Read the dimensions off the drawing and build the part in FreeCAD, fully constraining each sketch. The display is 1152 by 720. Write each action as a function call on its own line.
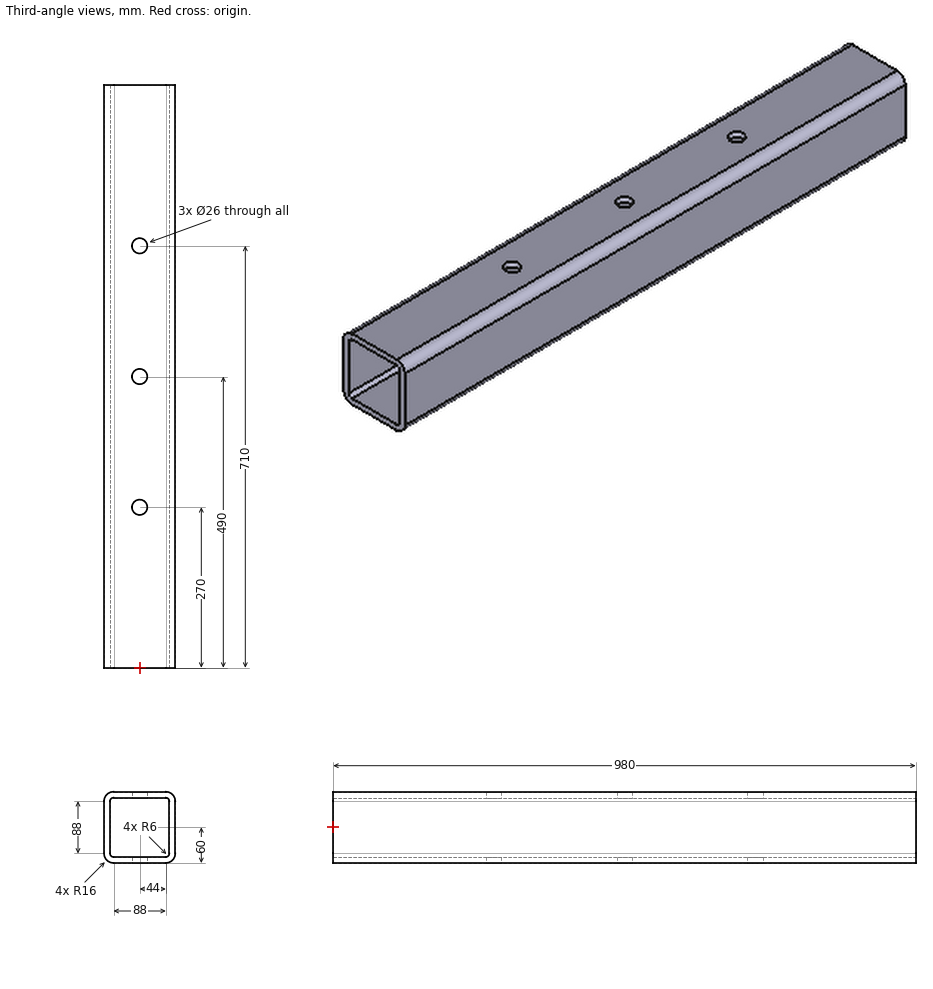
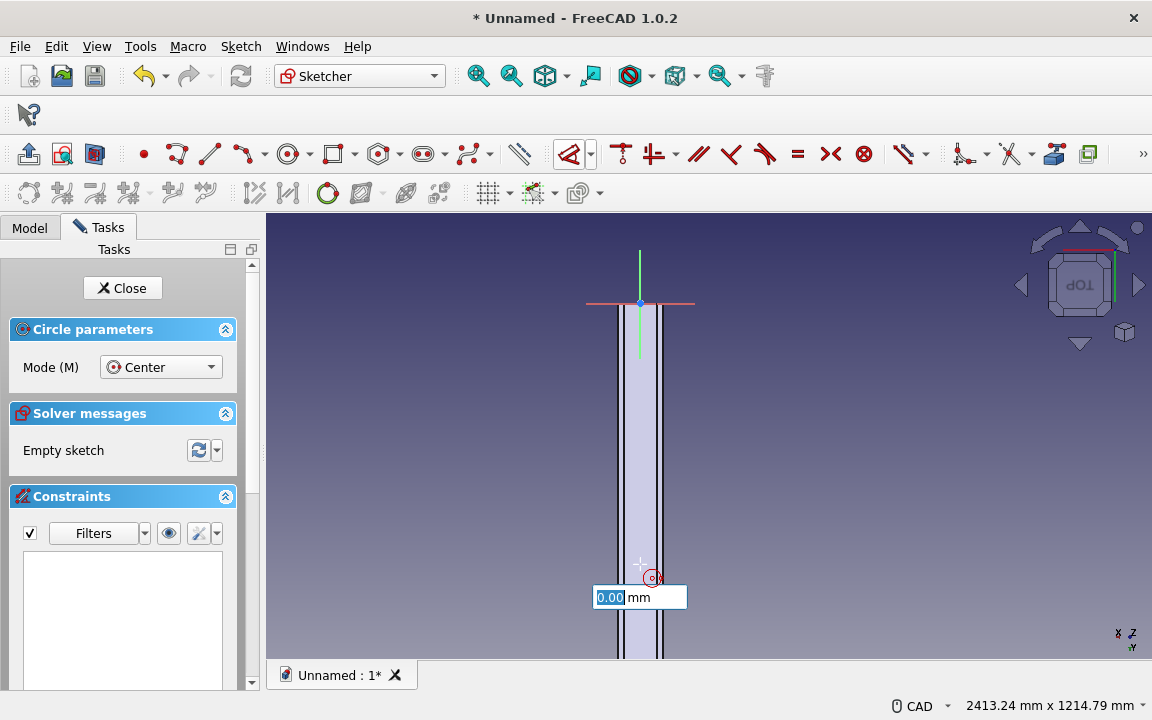
scroll(645, 563, up, 7)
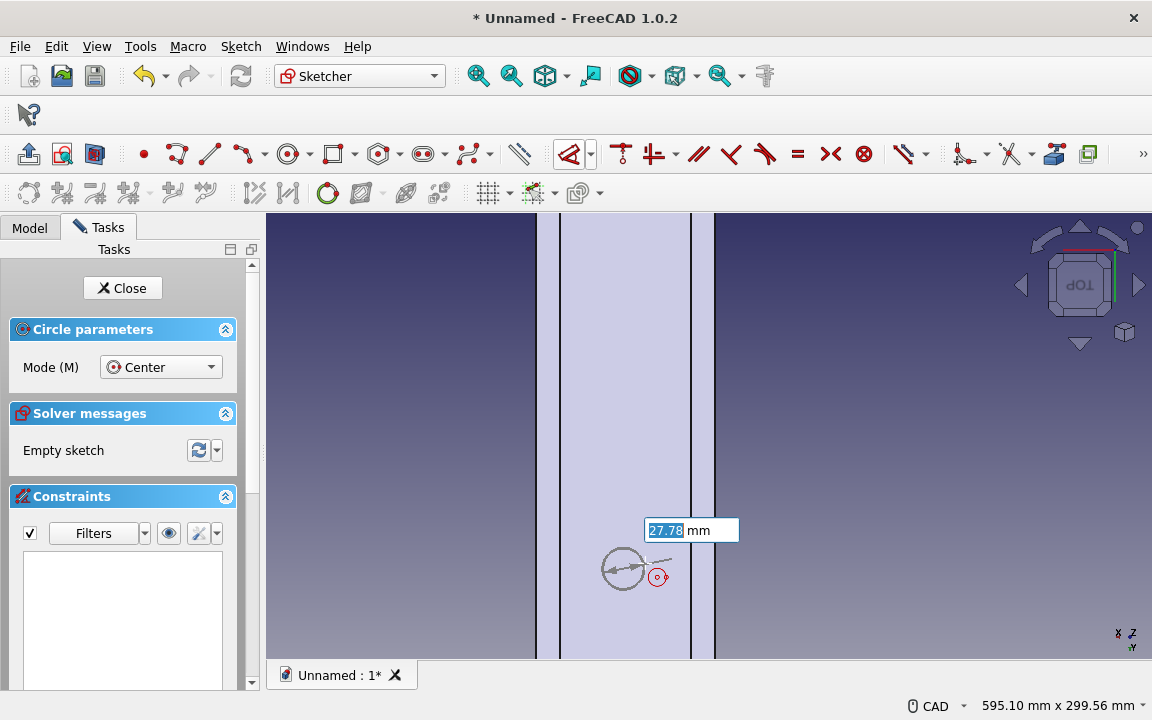
click(644, 559)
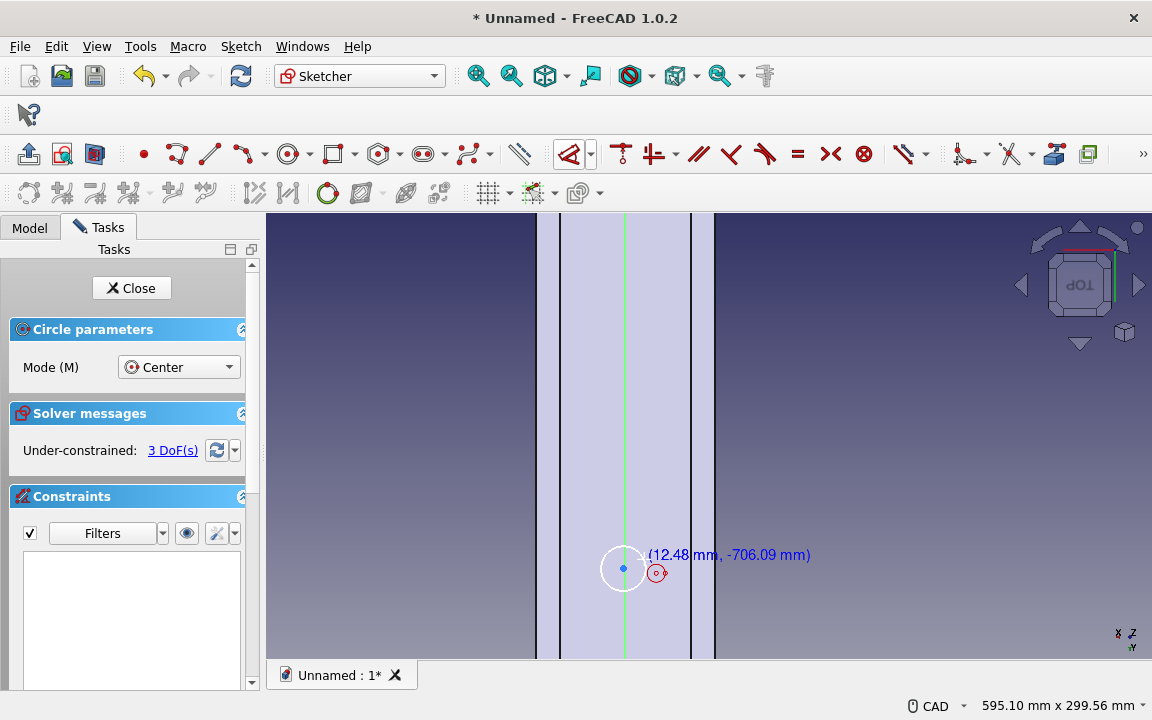
scroll(645, 563, down, 7)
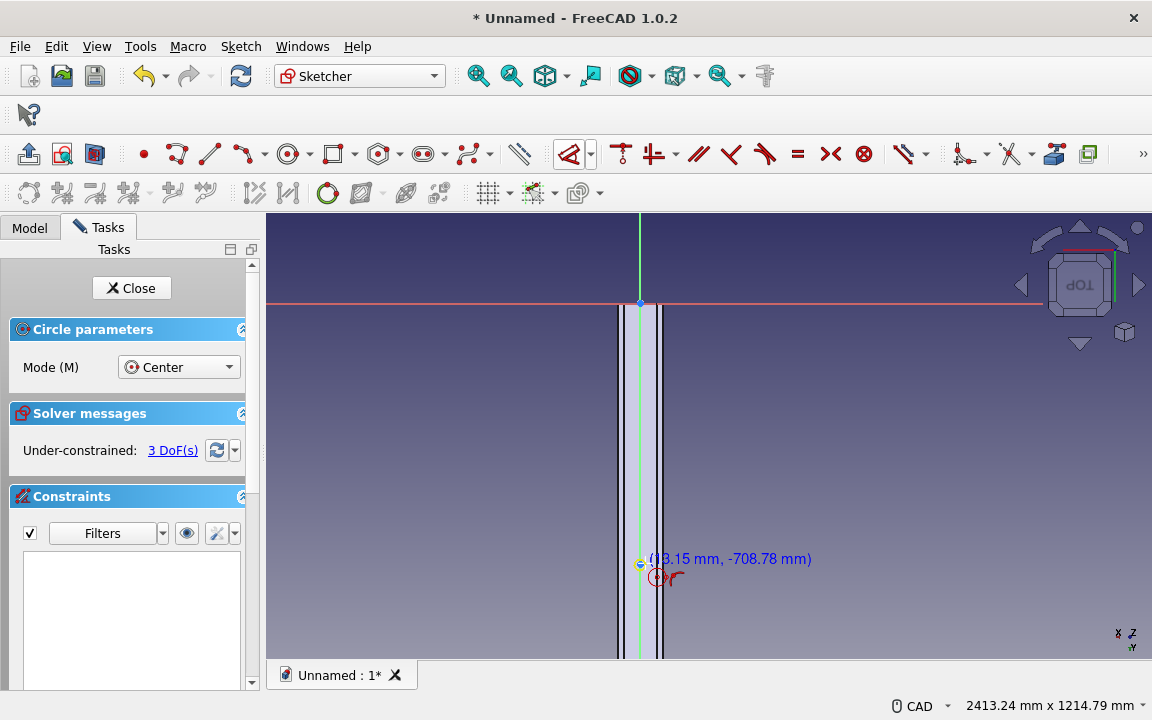
scroll(640, 484, up, 8)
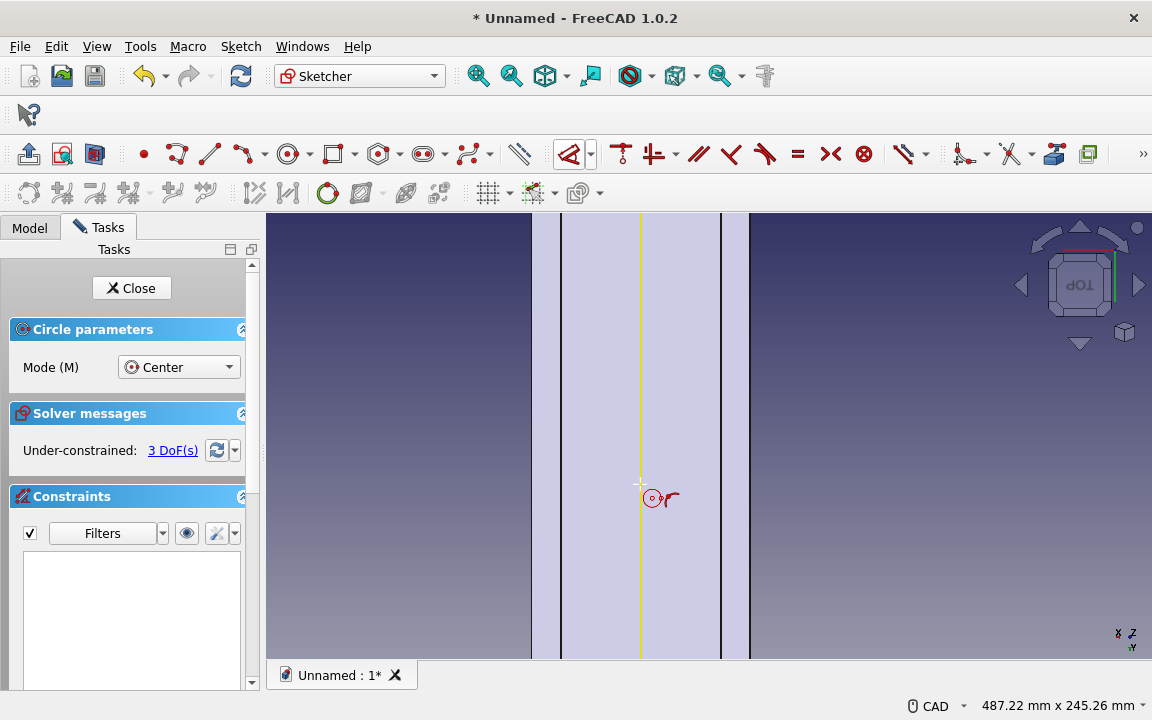
scroll(640, 484, down, 8)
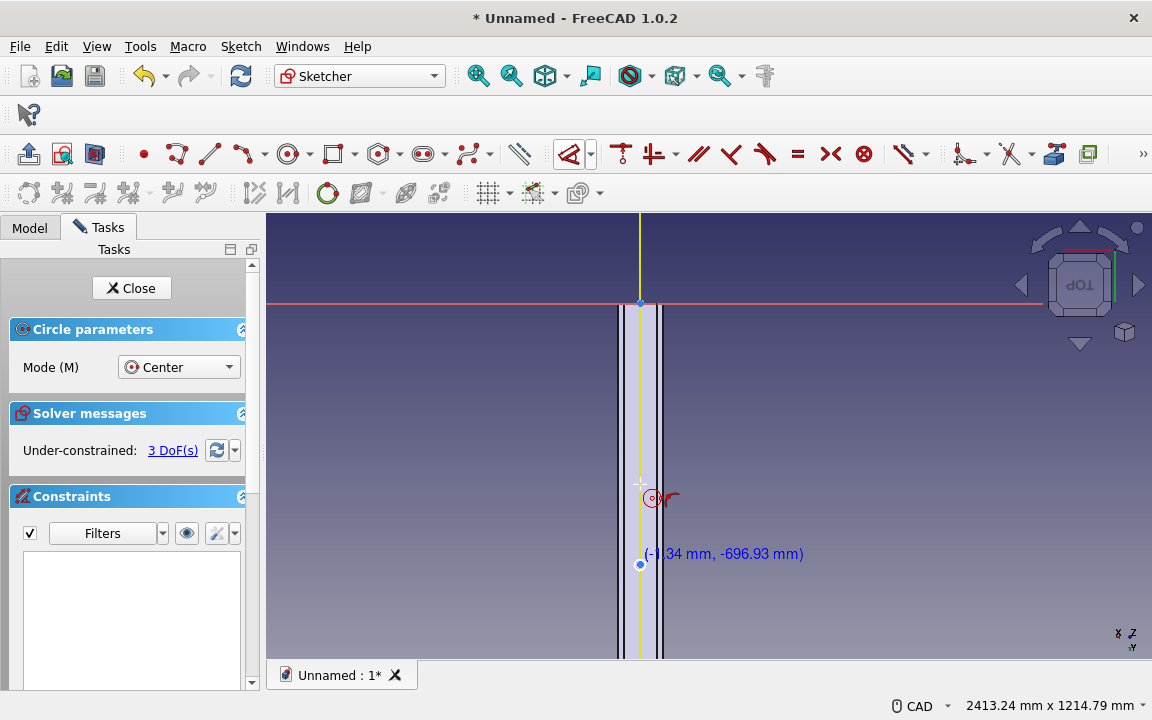
click(640, 484)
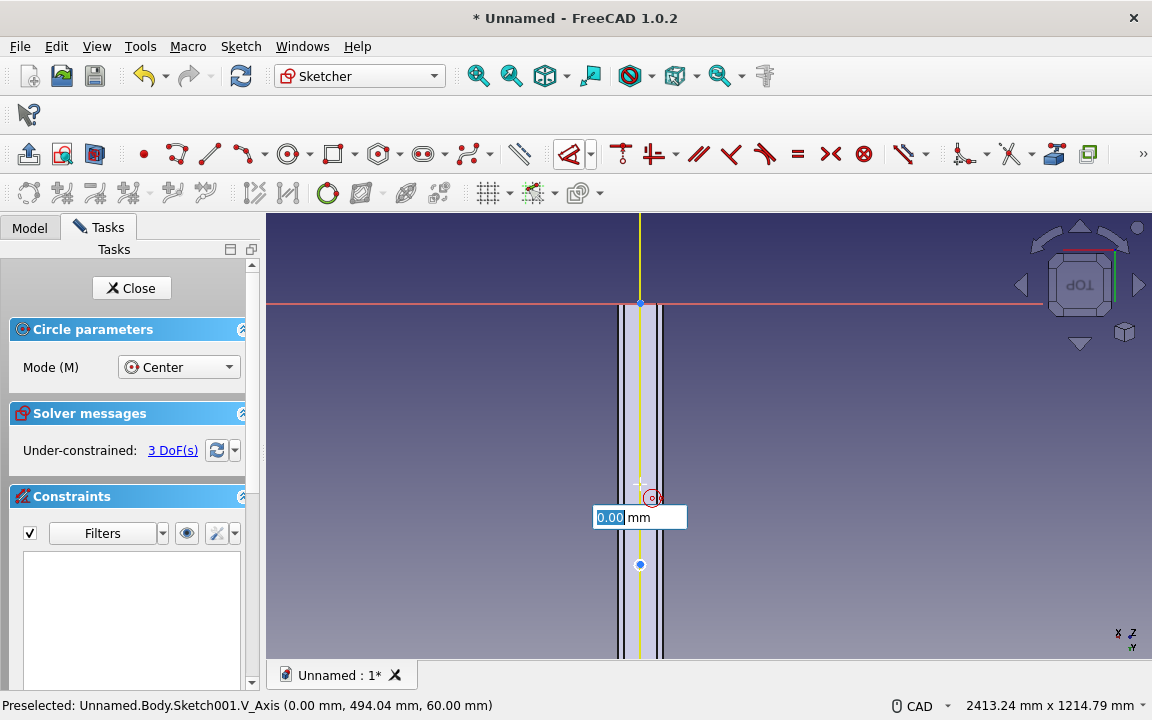
scroll(645, 482, up, 7)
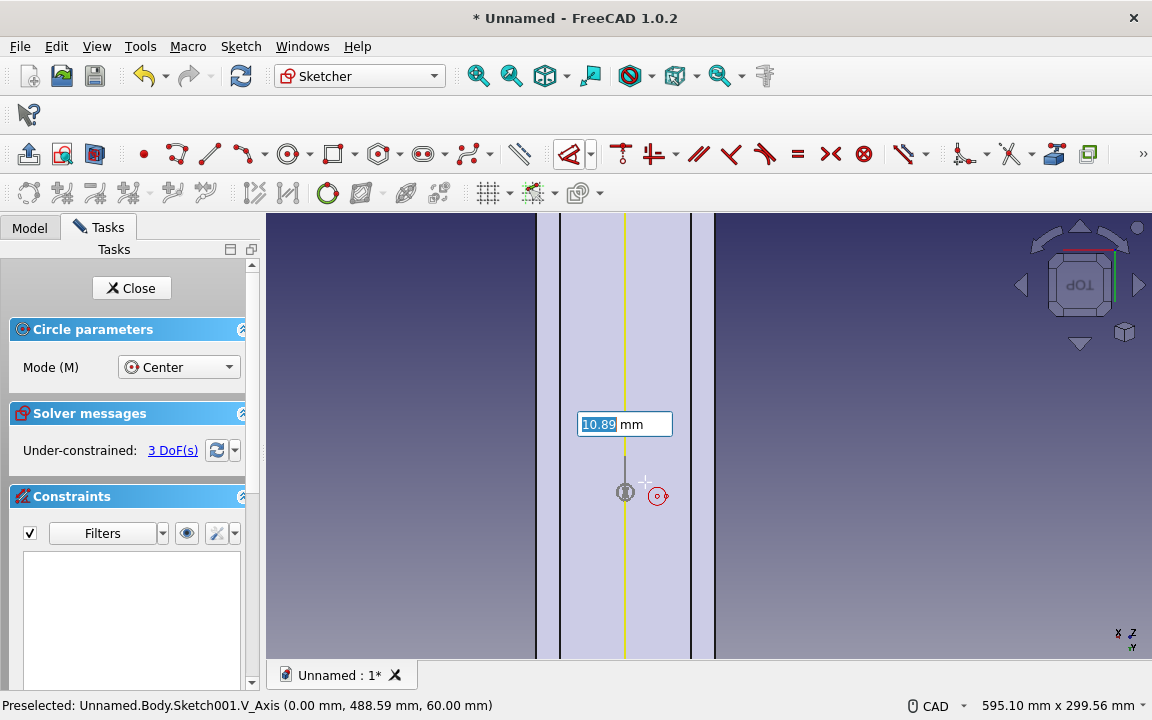
click(644, 480)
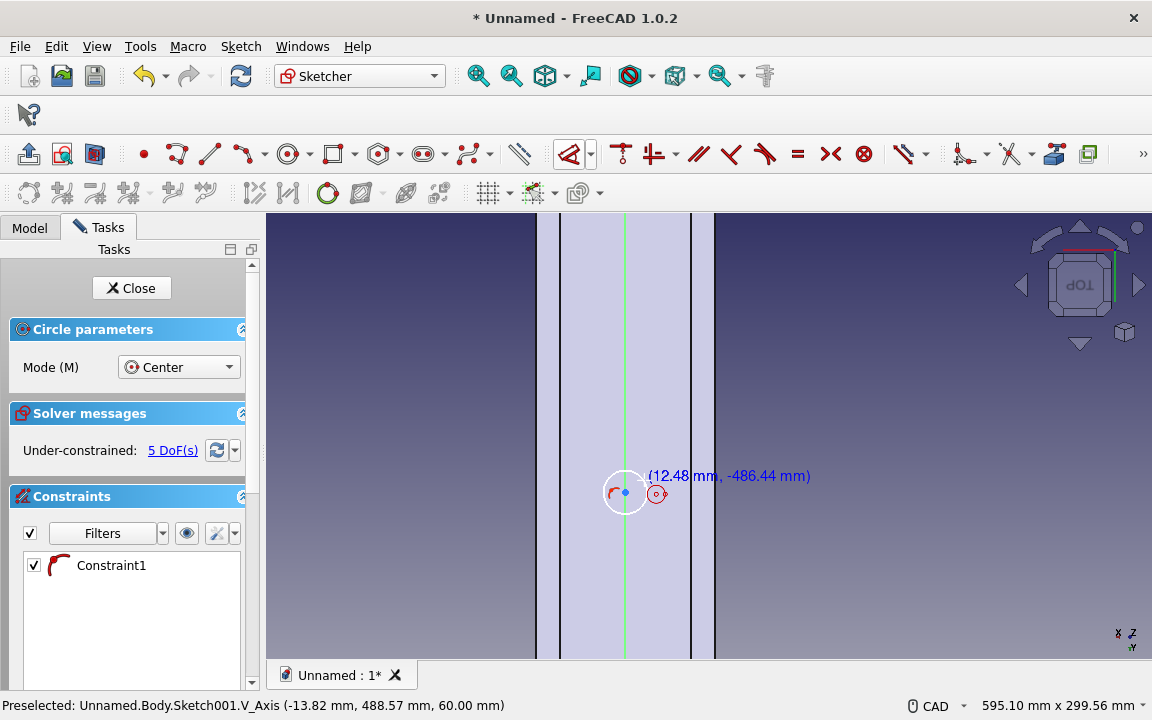
scroll(645, 482, down, 7)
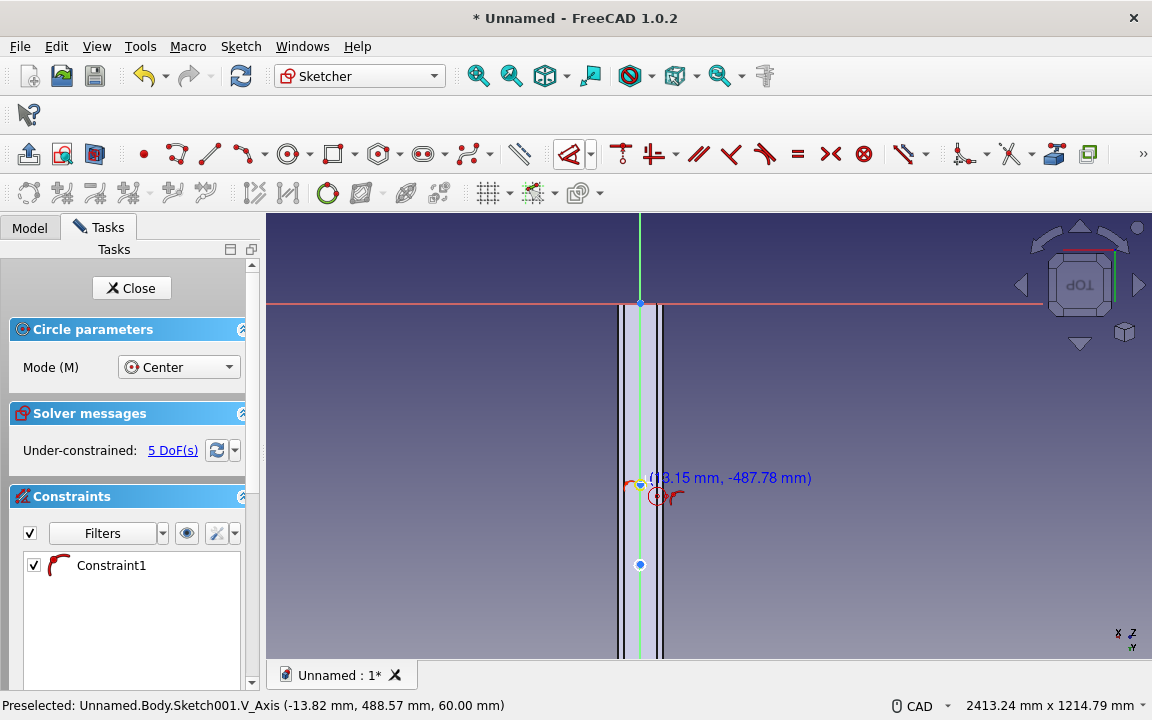
scroll(640, 403, up, 8)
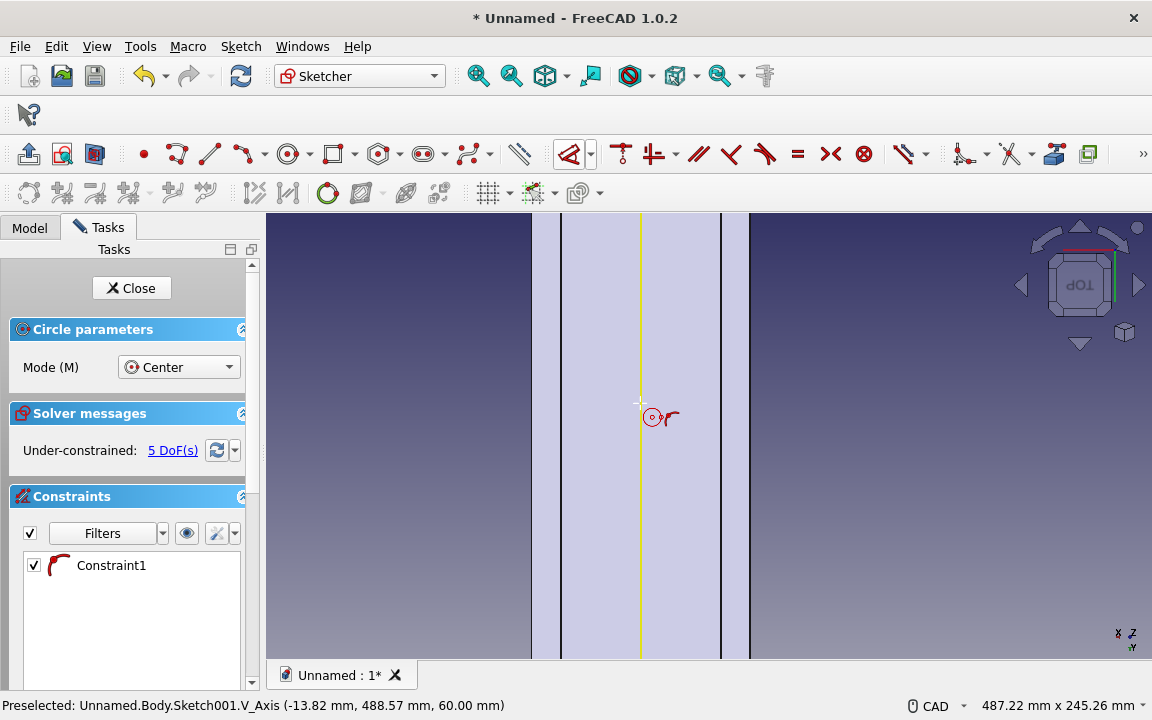
scroll(640, 403, down, 8)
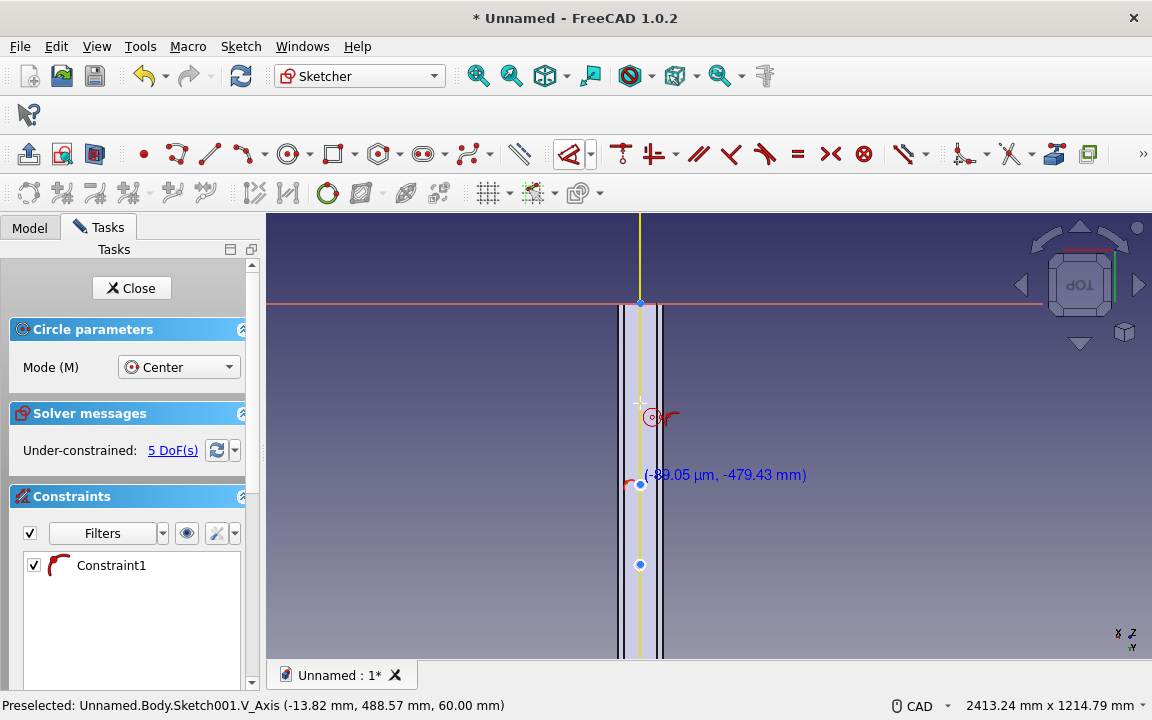
click(640, 403)